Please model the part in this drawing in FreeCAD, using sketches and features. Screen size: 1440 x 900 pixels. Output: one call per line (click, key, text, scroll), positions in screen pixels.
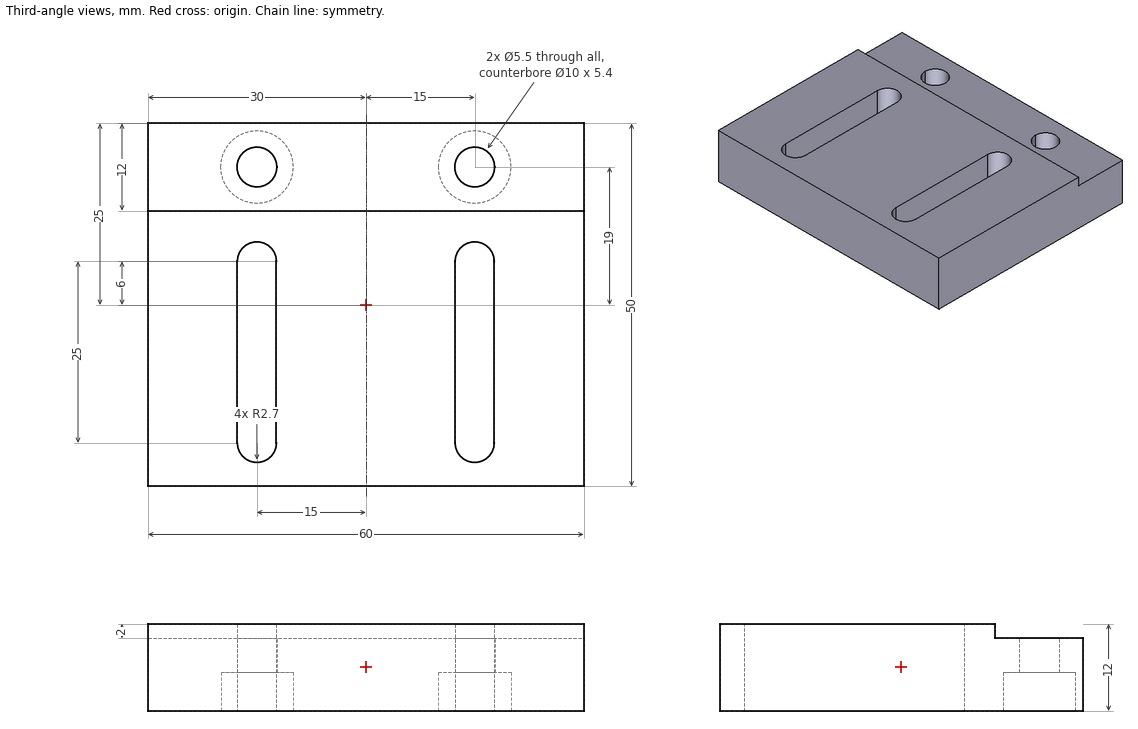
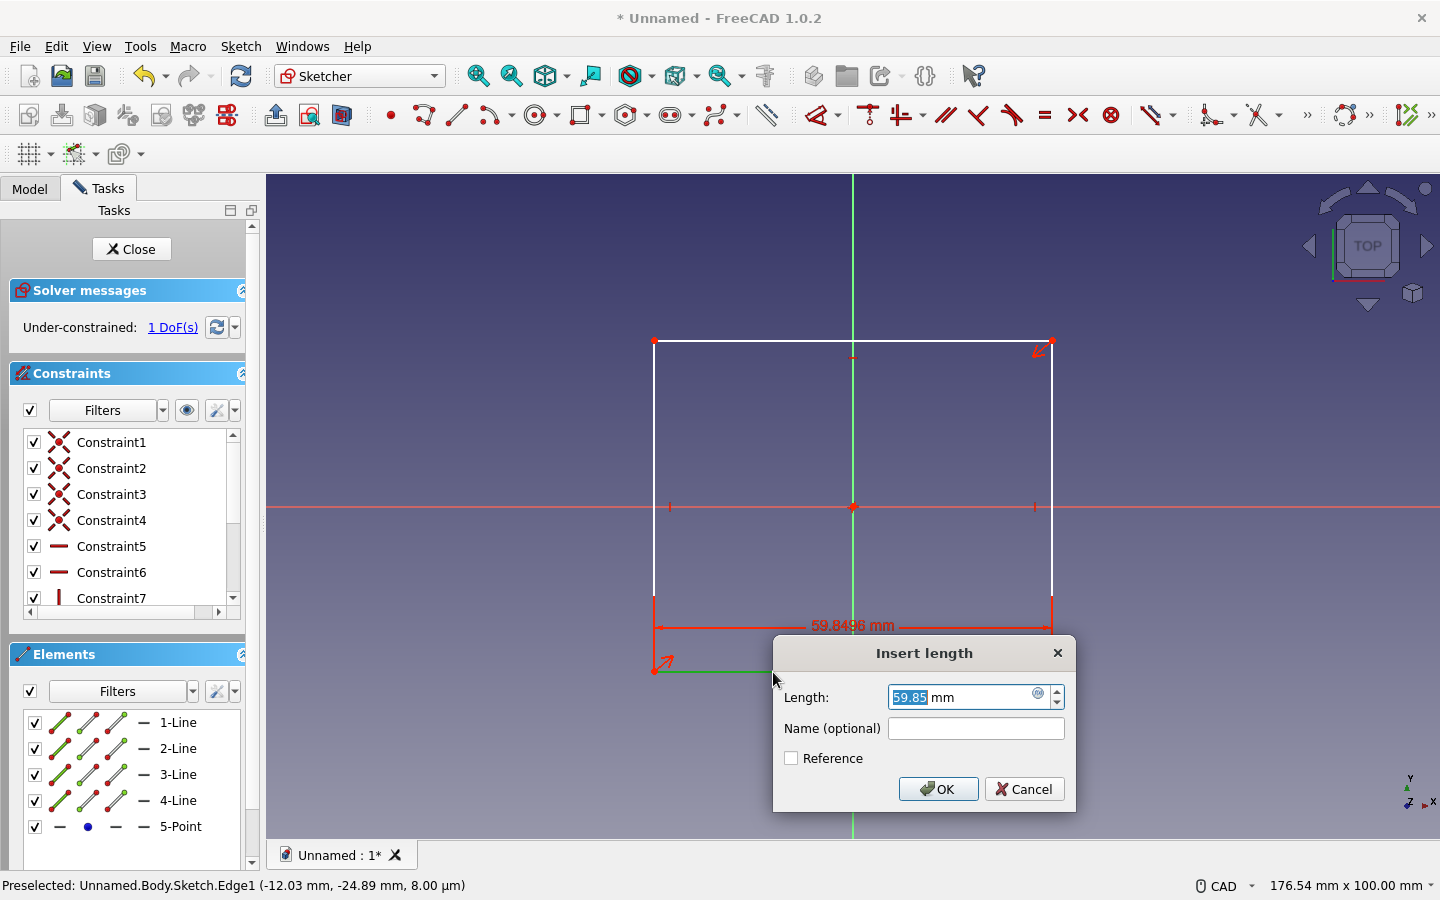
text(60)
key(Return)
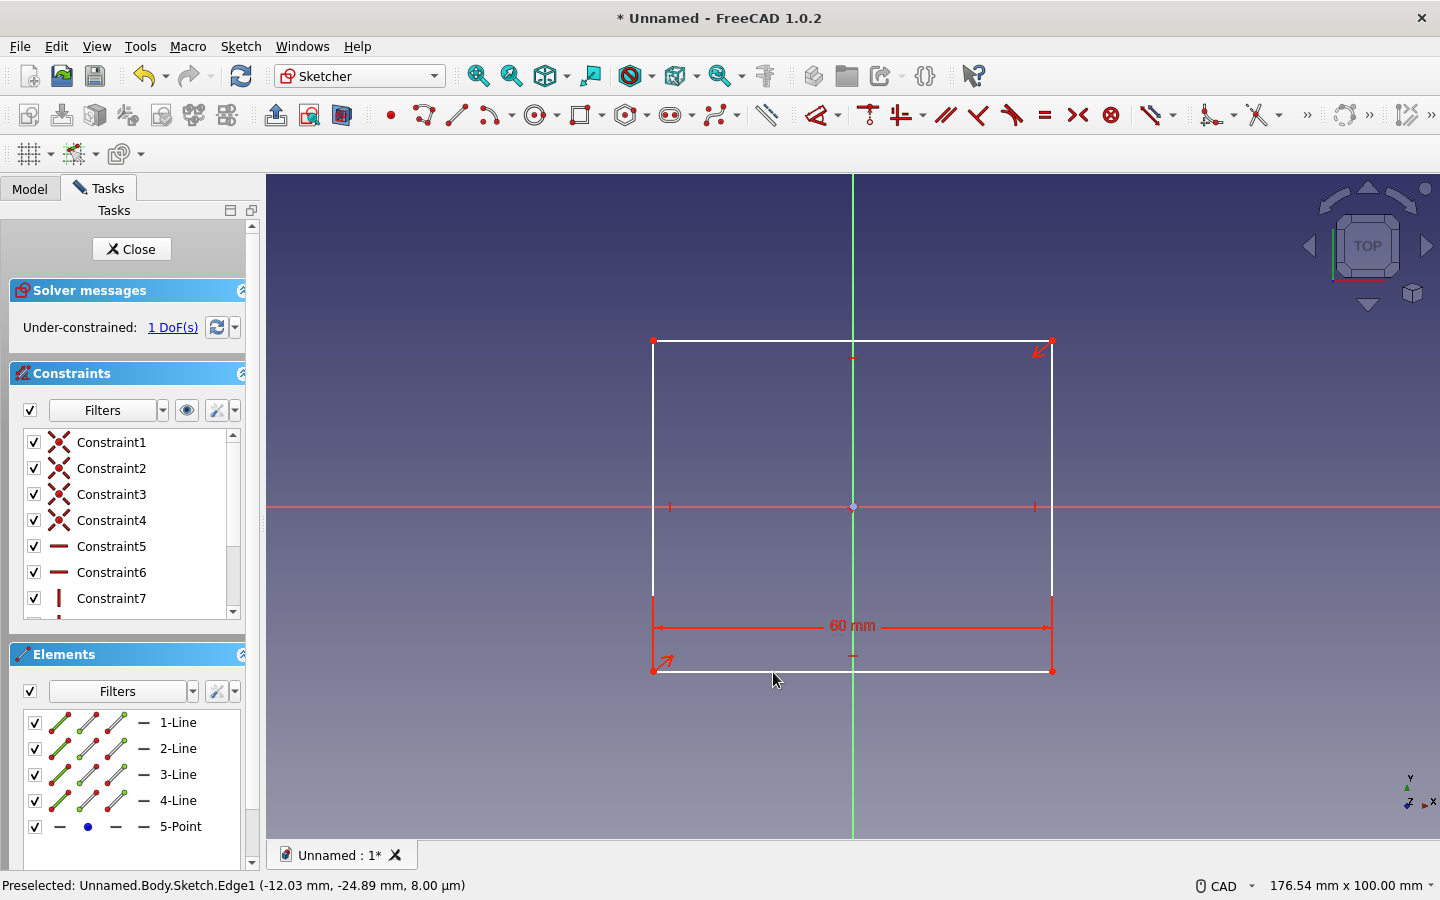
click(1052, 573)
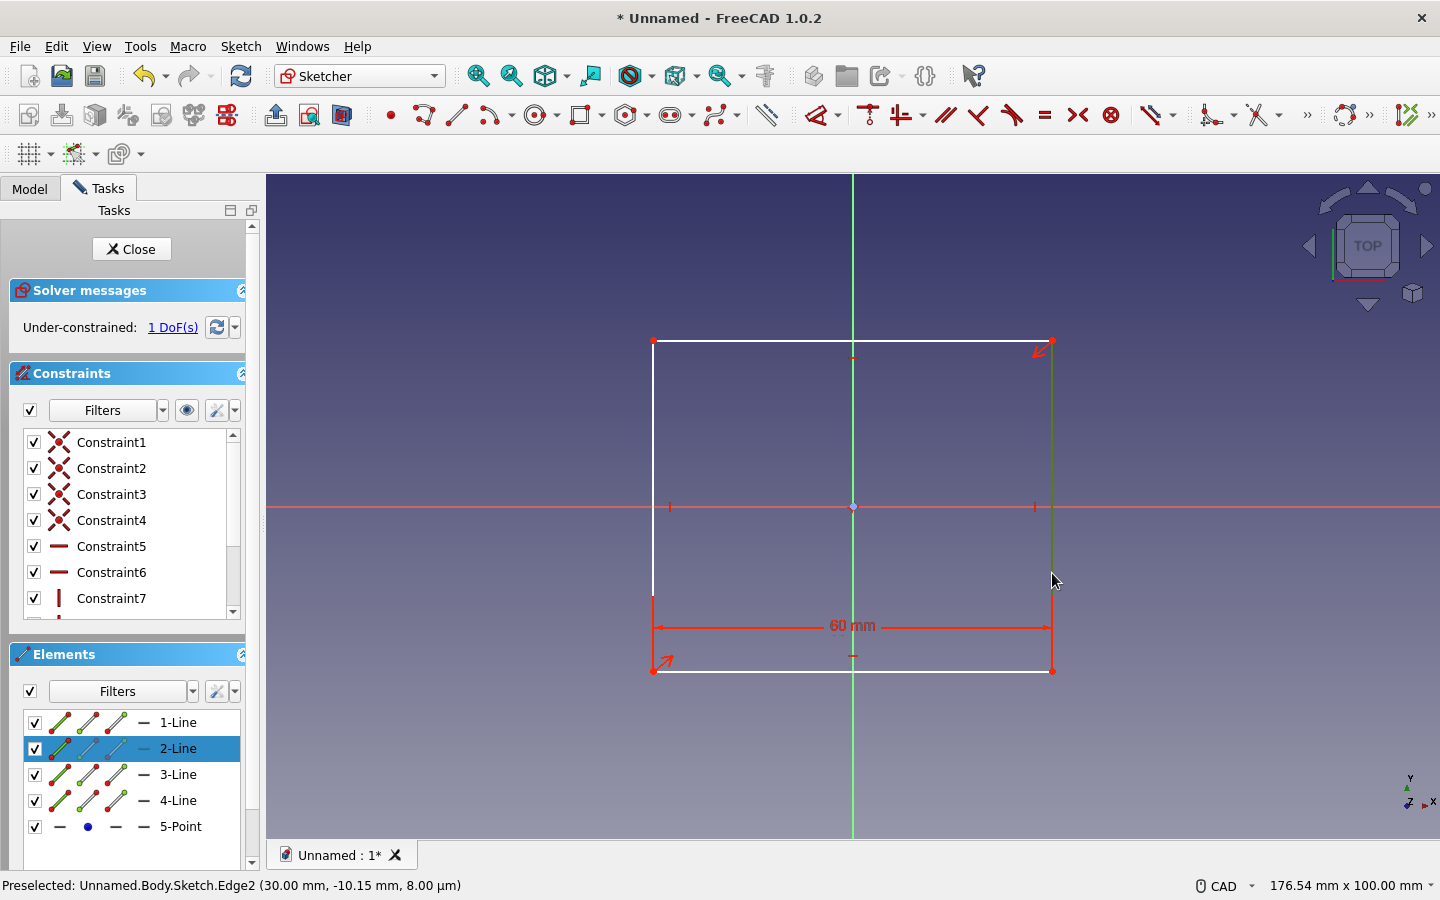
click(838, 116)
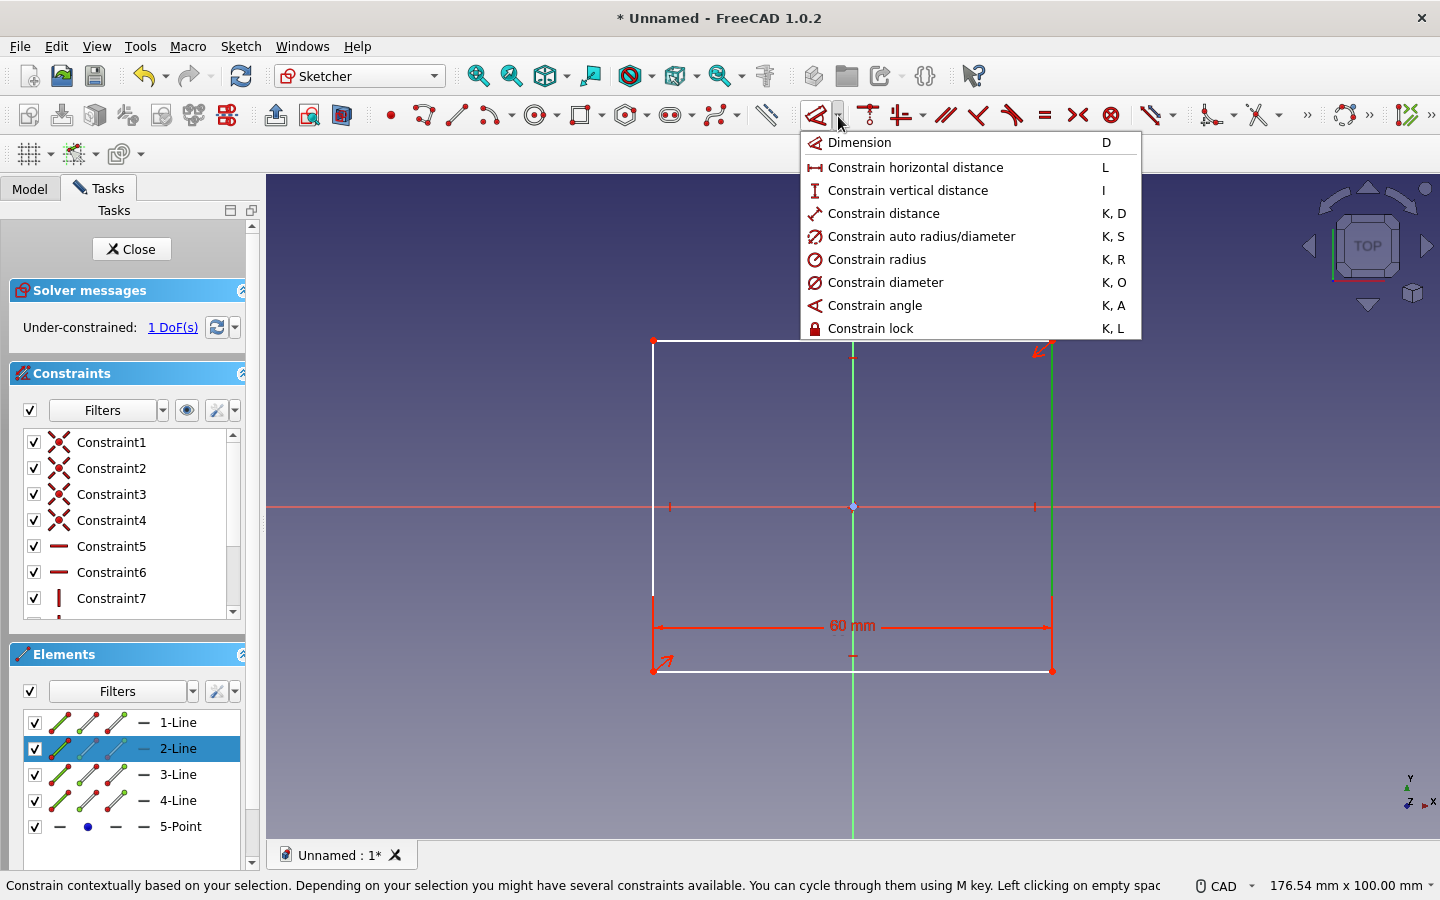
click(971, 190)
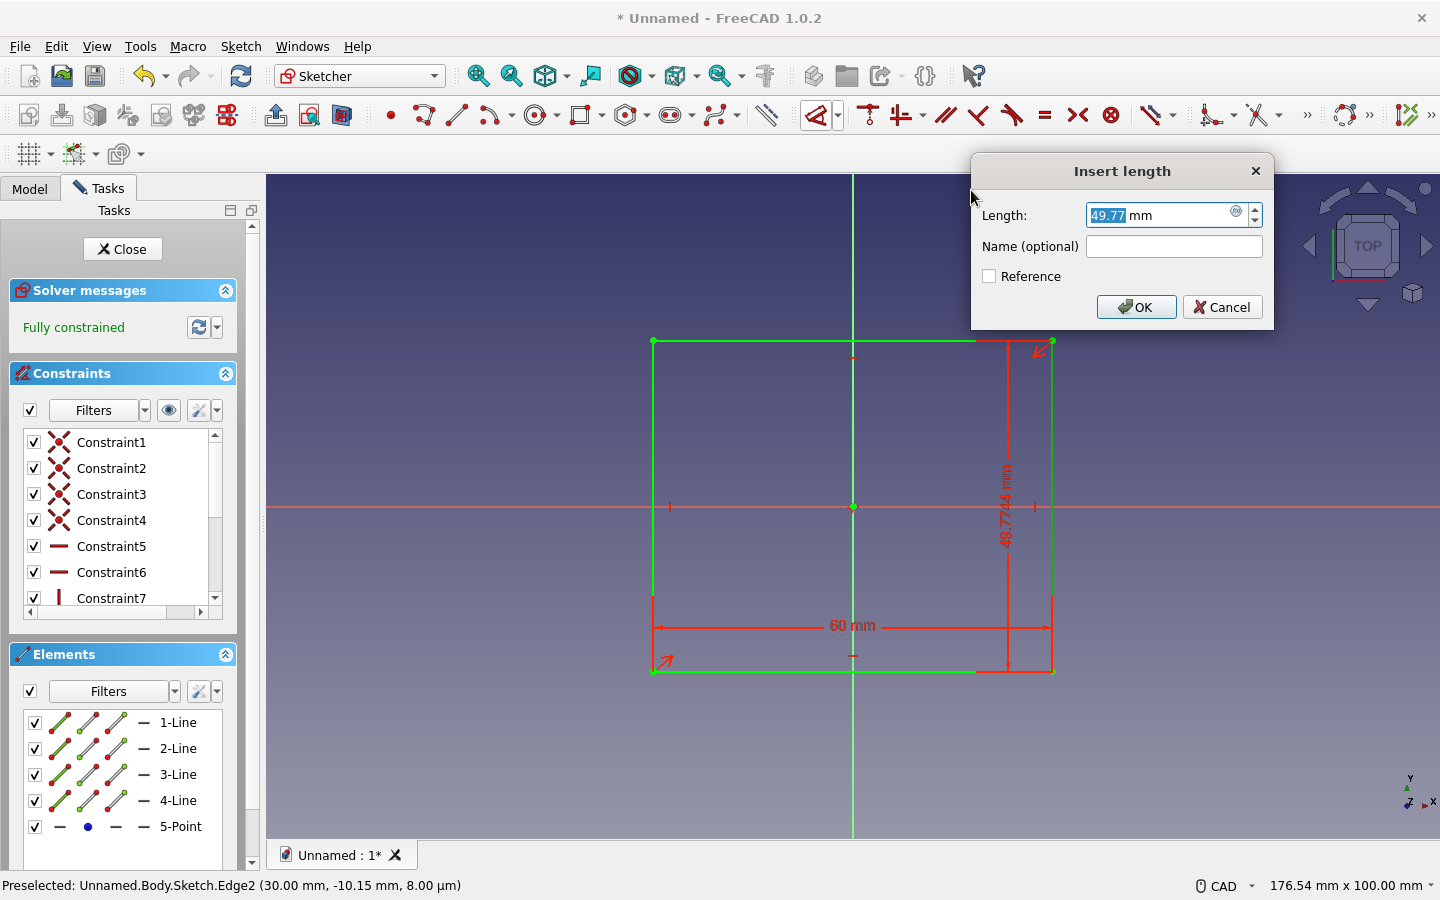
text(50)
key(Return)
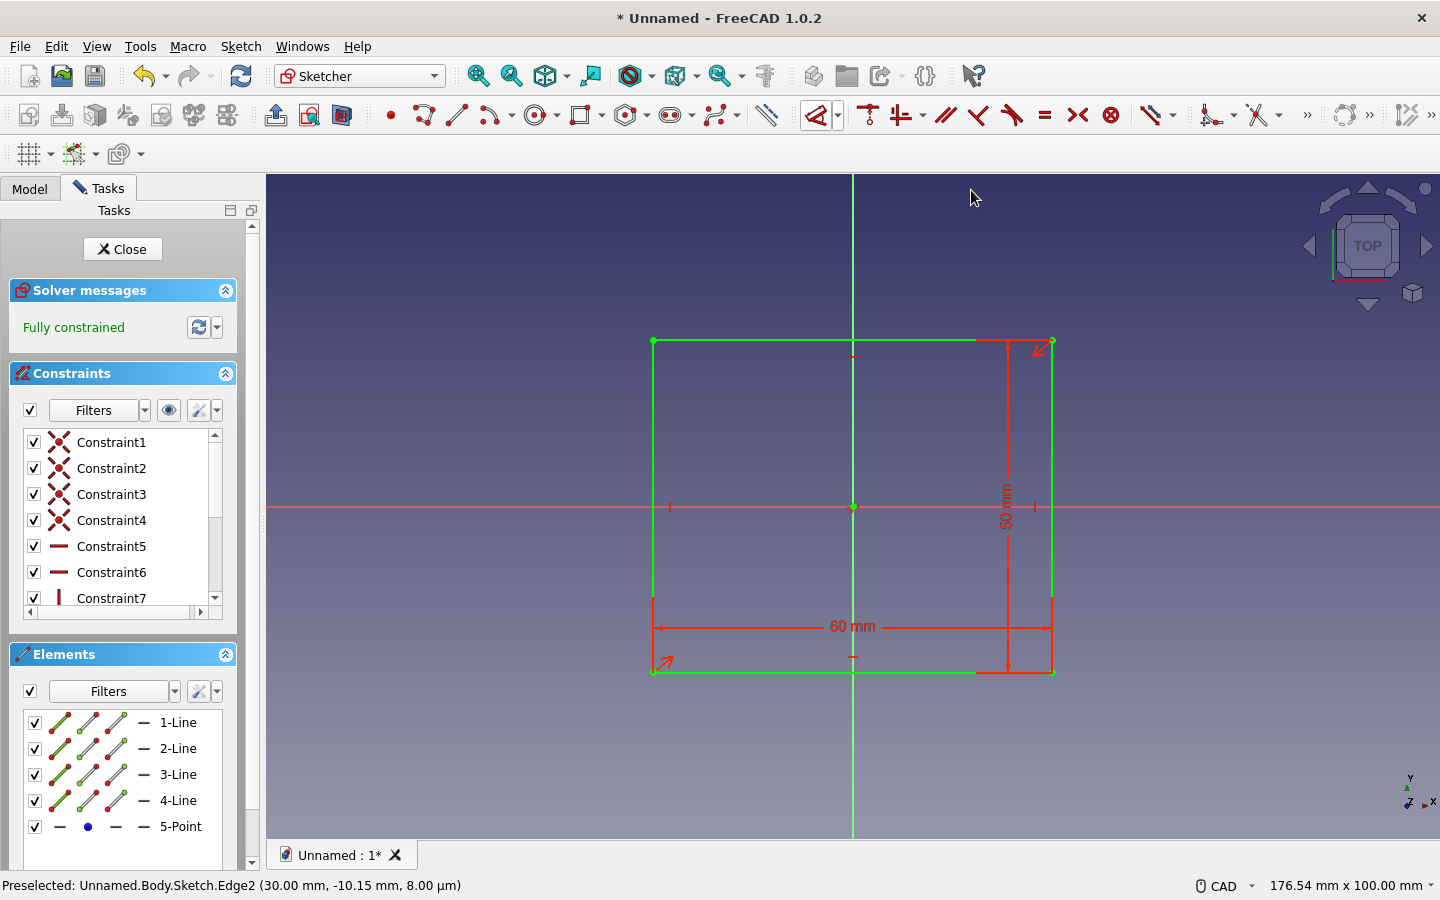
click(123, 249)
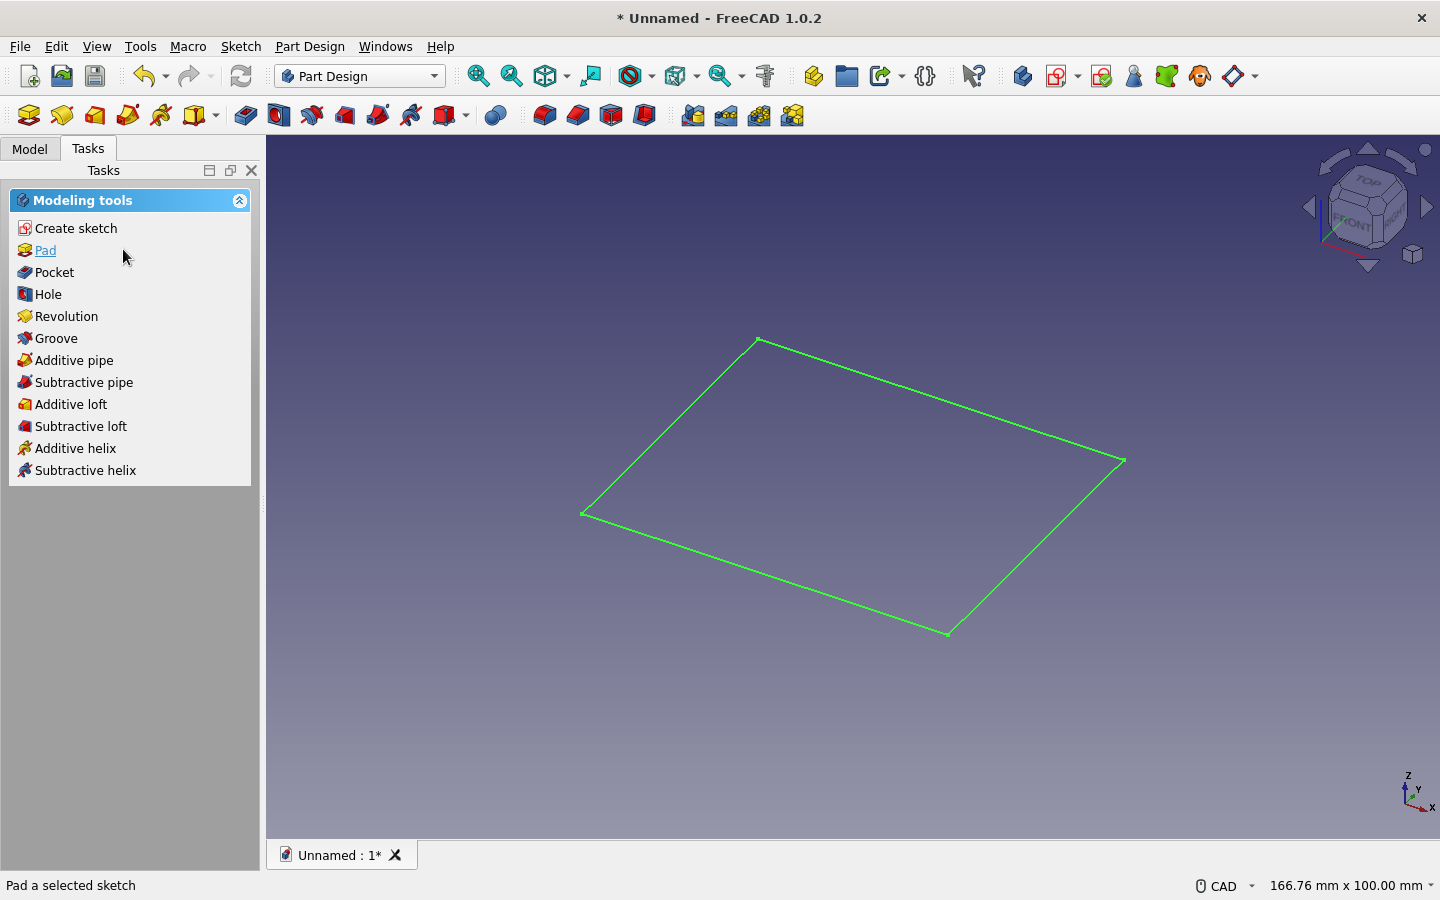
click(29, 116)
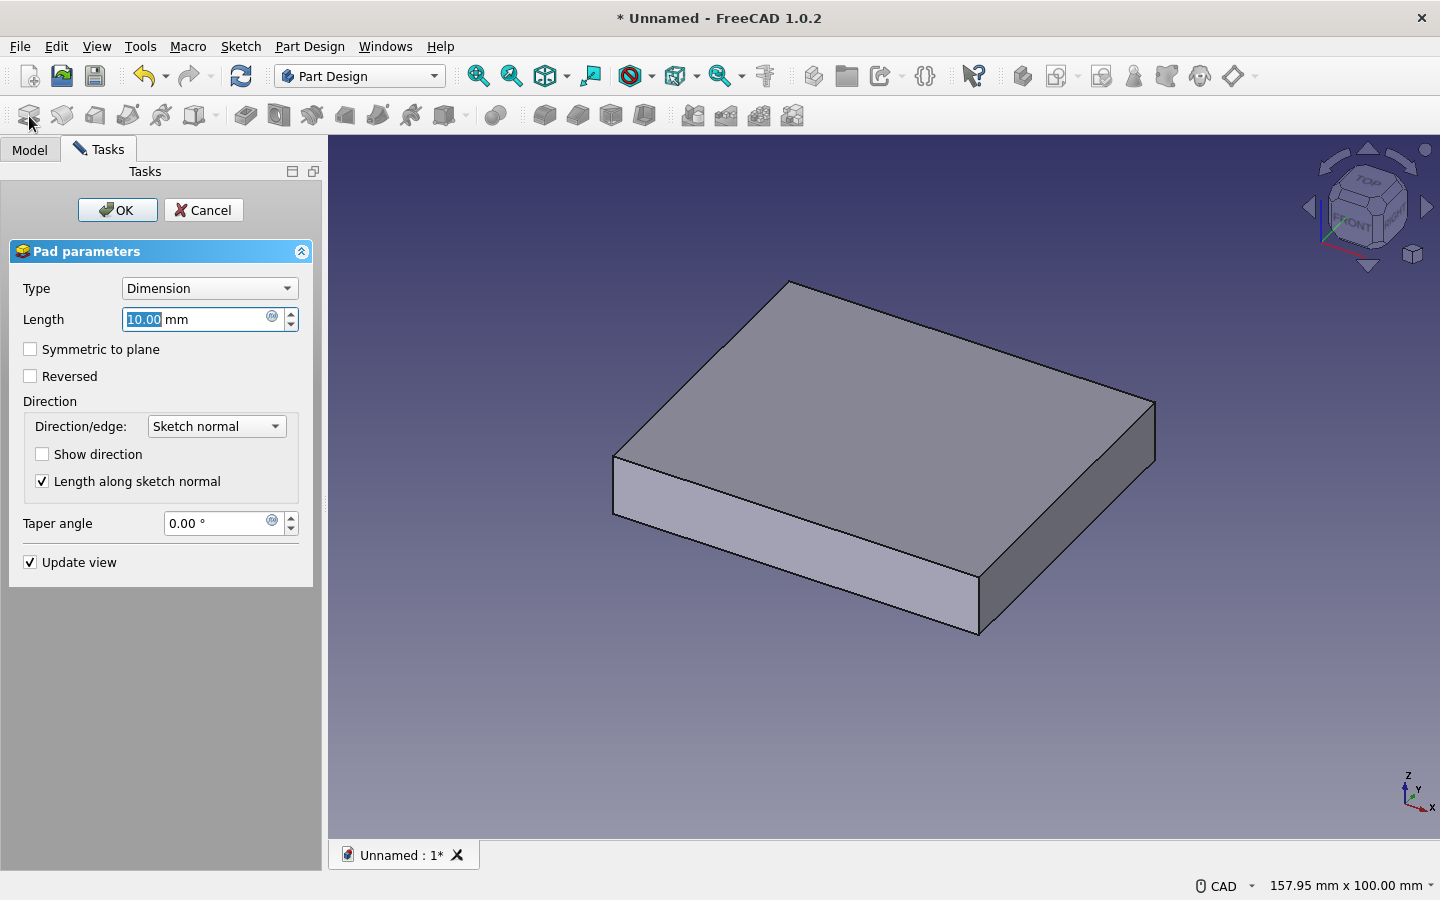
text(12)
key(Tab)